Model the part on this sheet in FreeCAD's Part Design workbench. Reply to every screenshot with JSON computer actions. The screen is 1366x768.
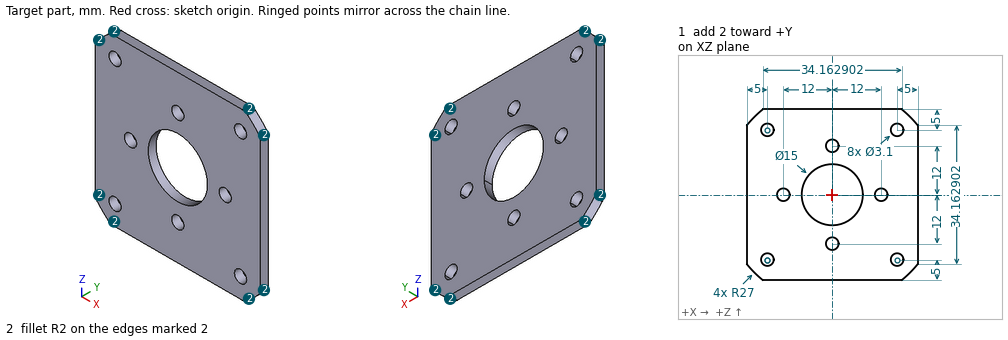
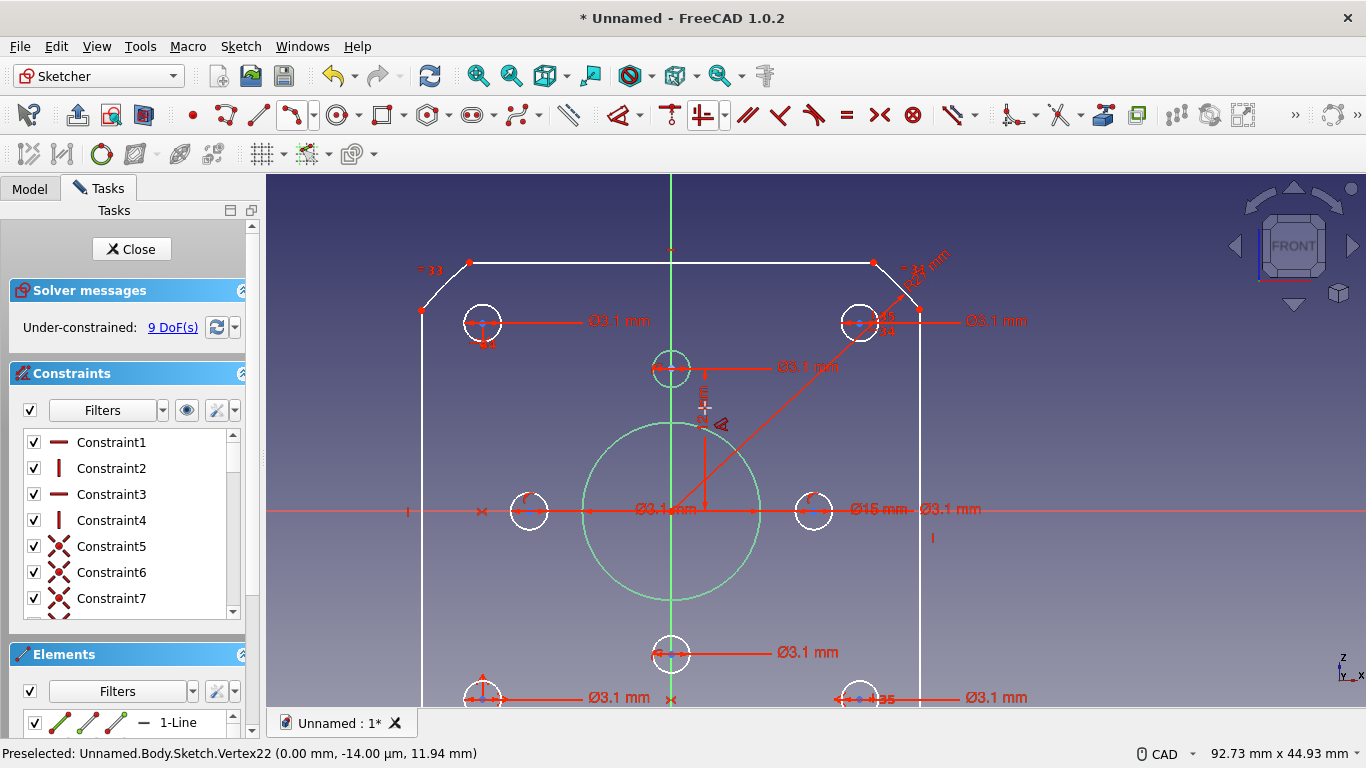
{"action": "left_click", "coordinate": [814, 511]}
{"action": "left_click", "coordinate": [710, 545]}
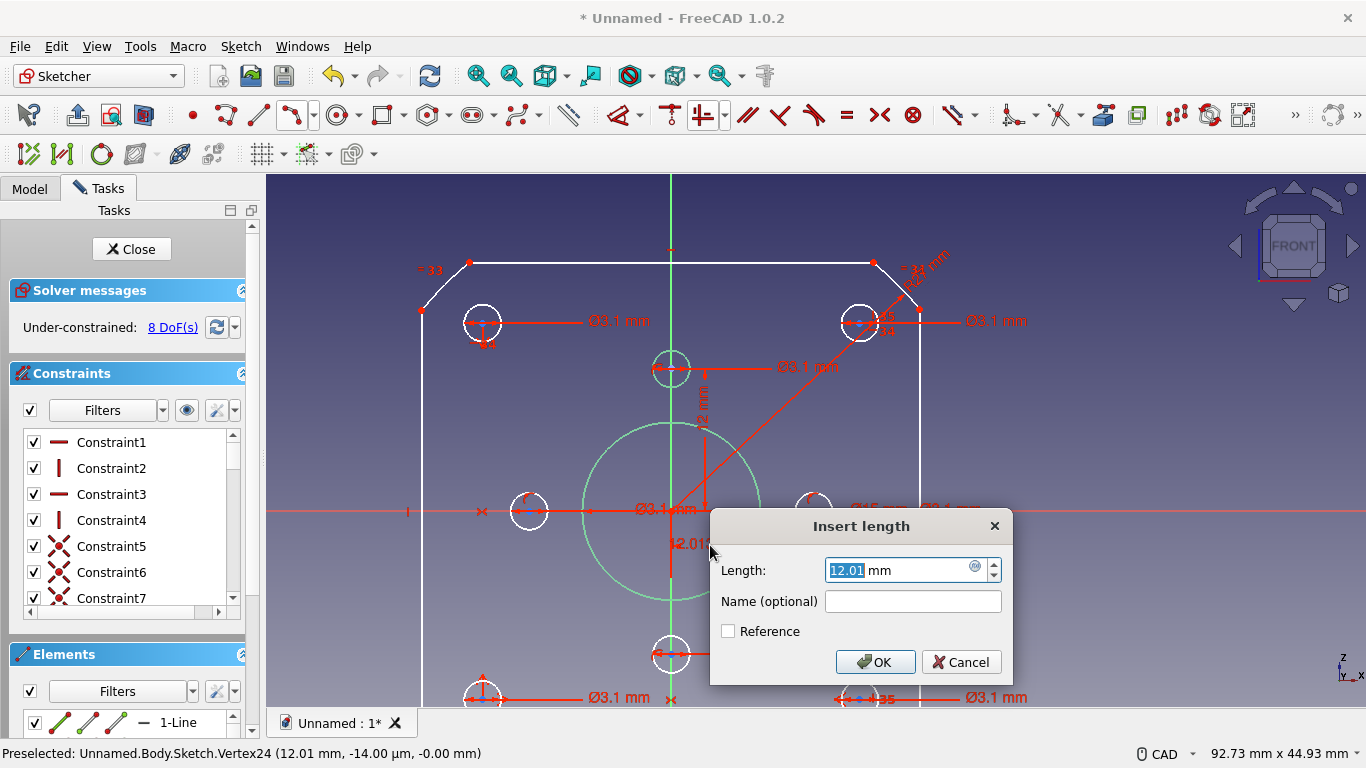
{"action": "type", "text": "12"}
{"action": "key", "text": "Return"}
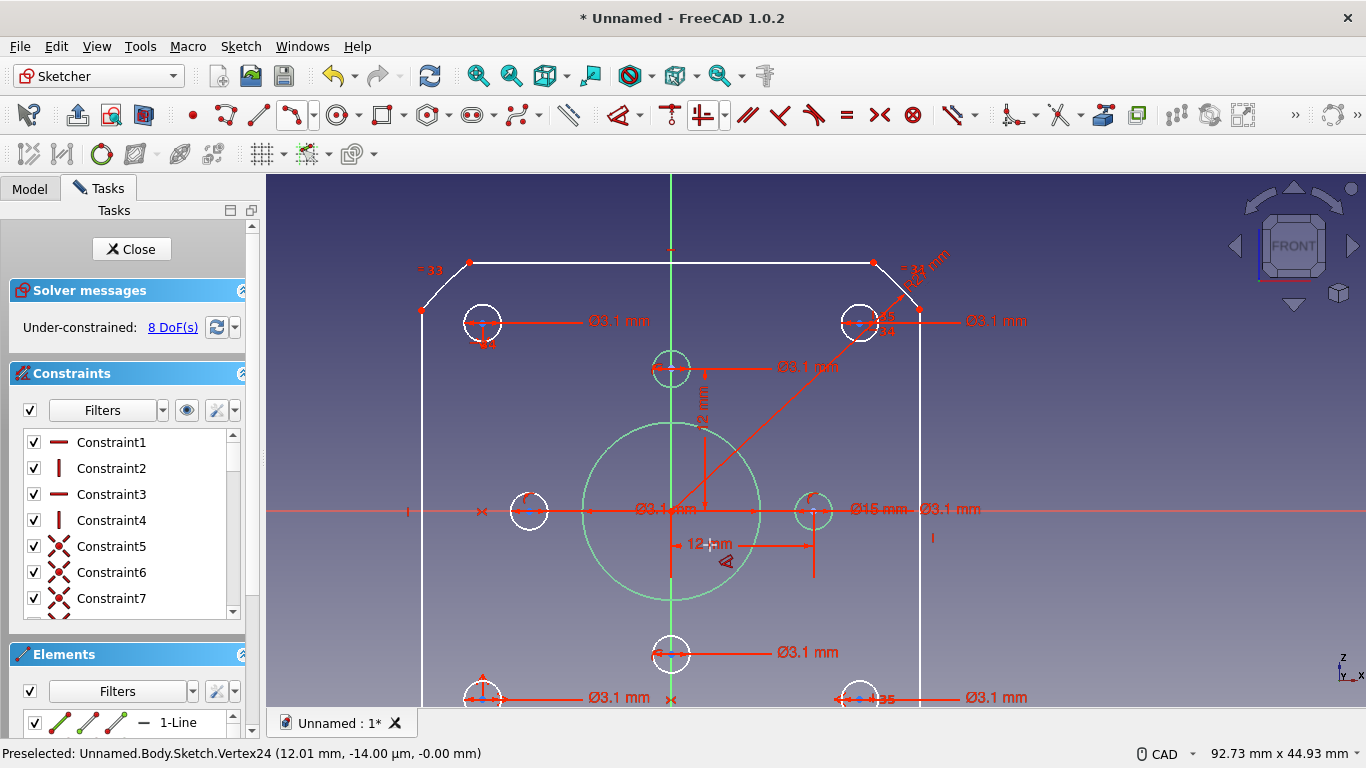
{"action": "left_click", "coordinate": [529, 511]}
{"action": "left_click", "coordinate": [568, 545]}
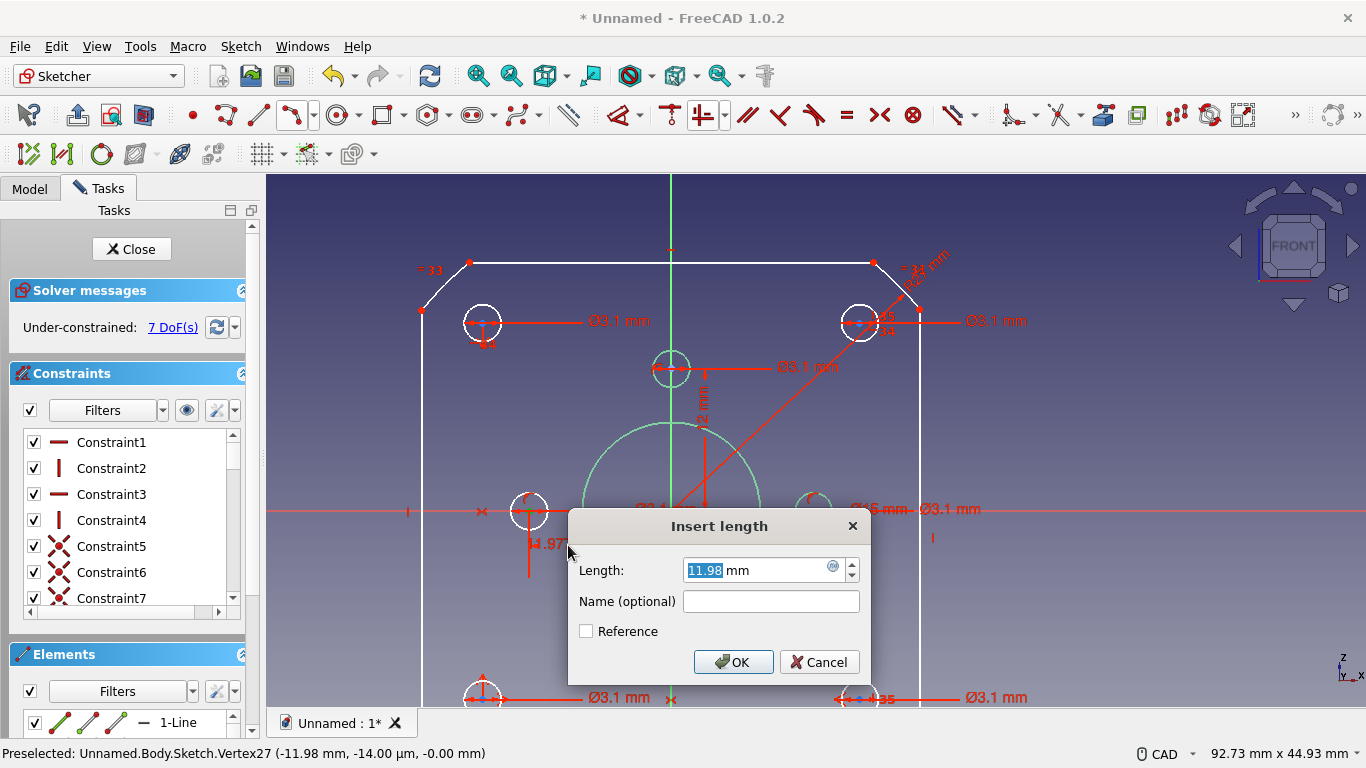
{"action": "type", "text": "12"}
{"action": "key", "text": "Return"}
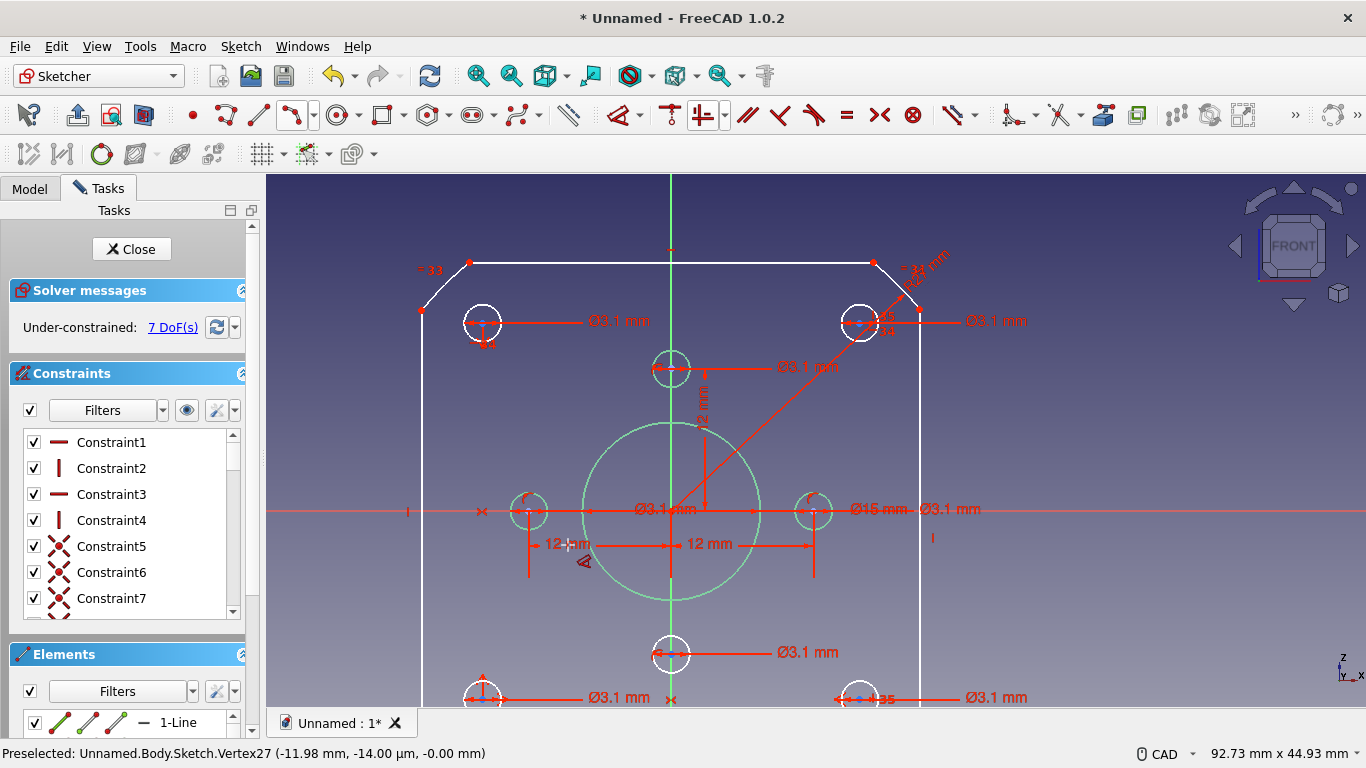
{"action": "left_click", "coordinate": [671, 654]}
{"action": "left_click", "coordinate": [705, 616]}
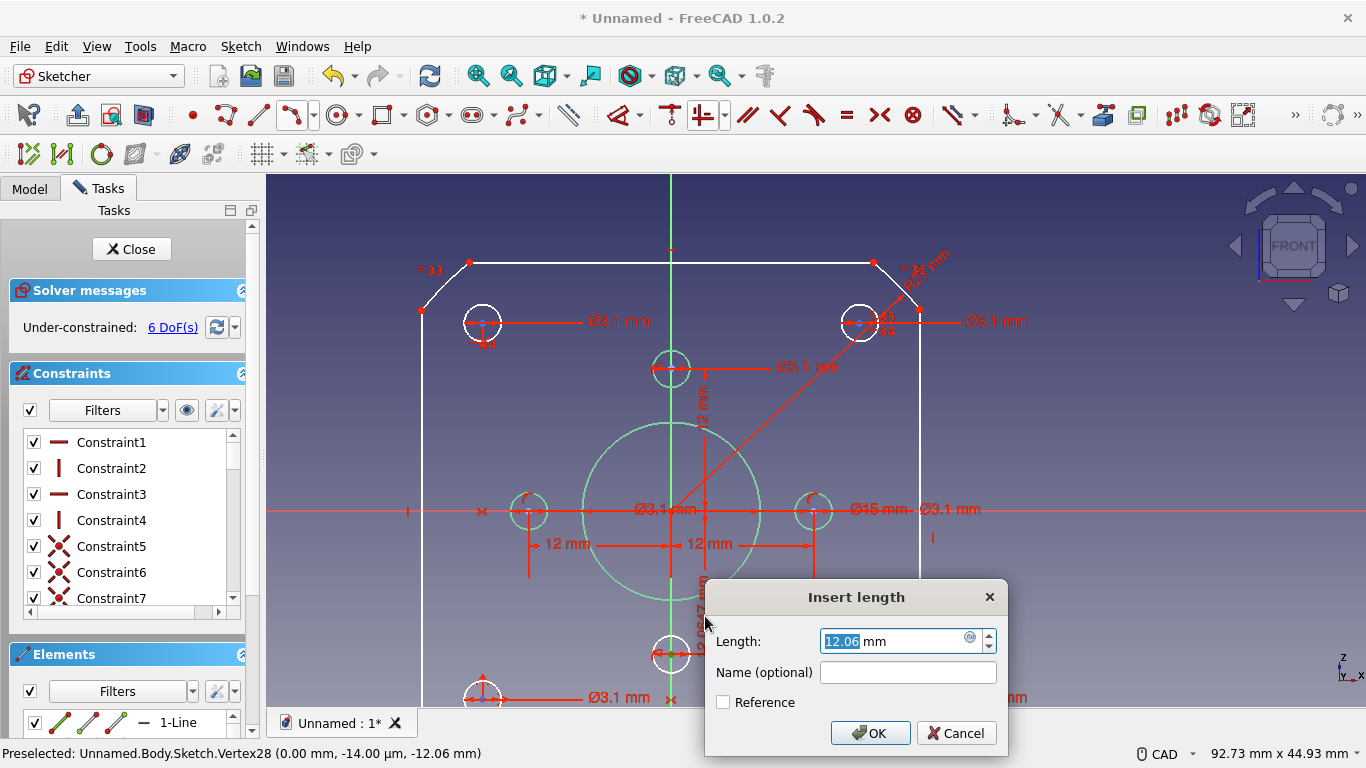
{"action": "type", "text": "12"}
{"action": "key", "text": "Return"}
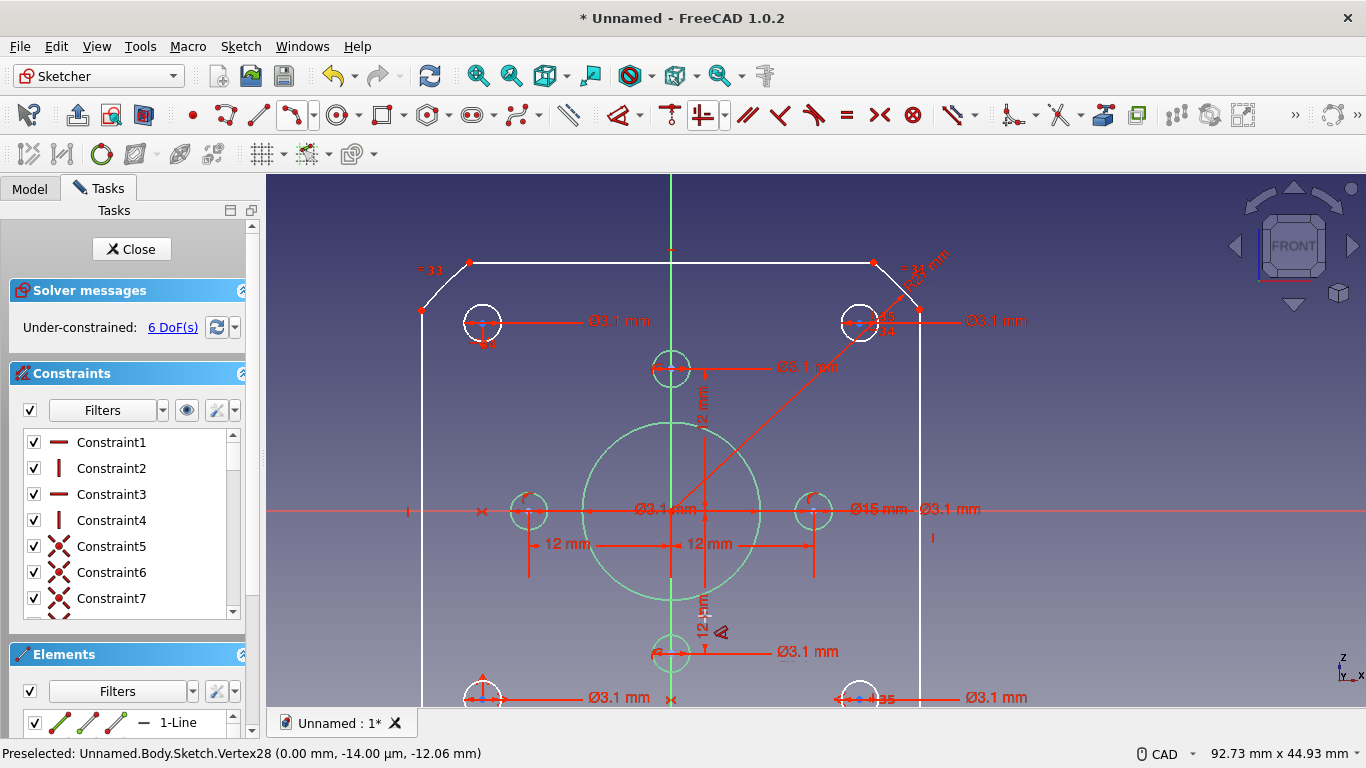
{"action": "left_click", "coordinate": [920, 309]}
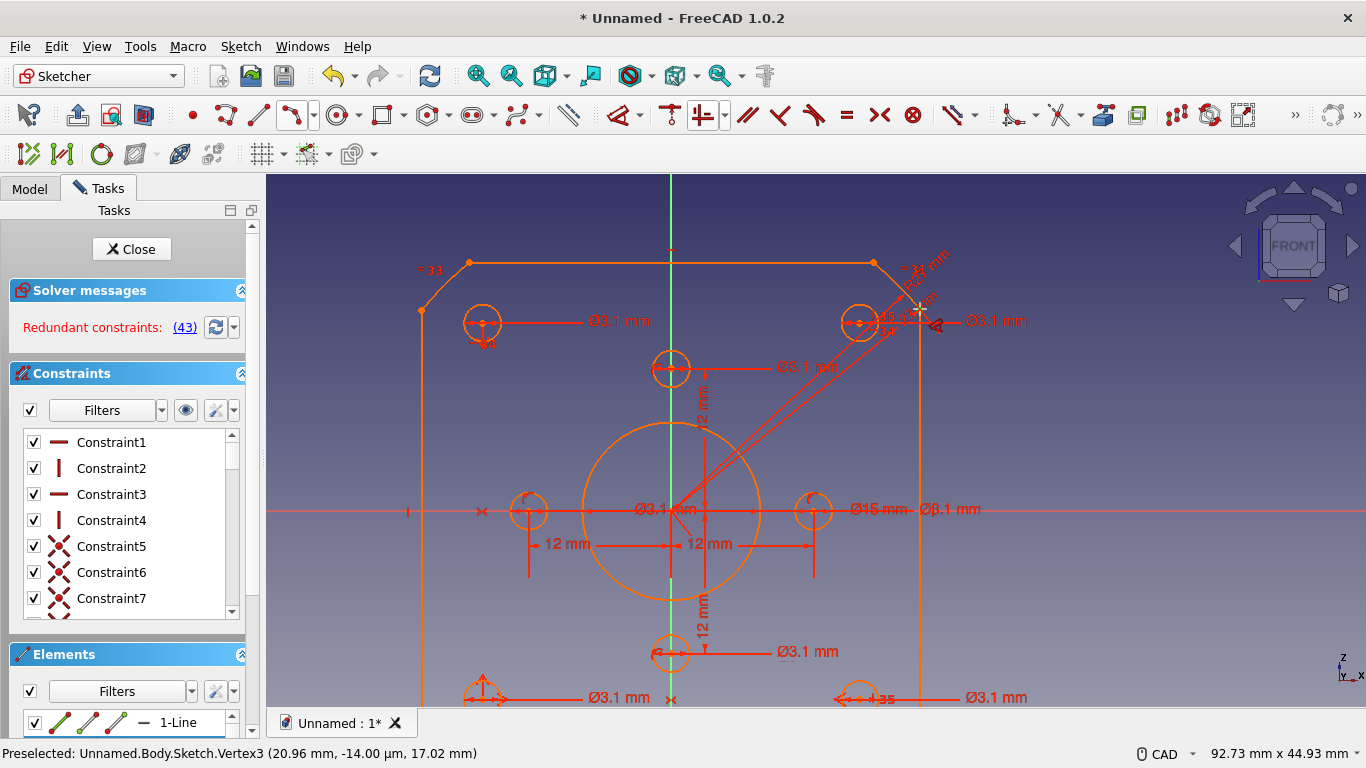
{"action": "left_click", "coordinate": [860, 323]}
{"action": "left_click", "coordinate": [890, 357]}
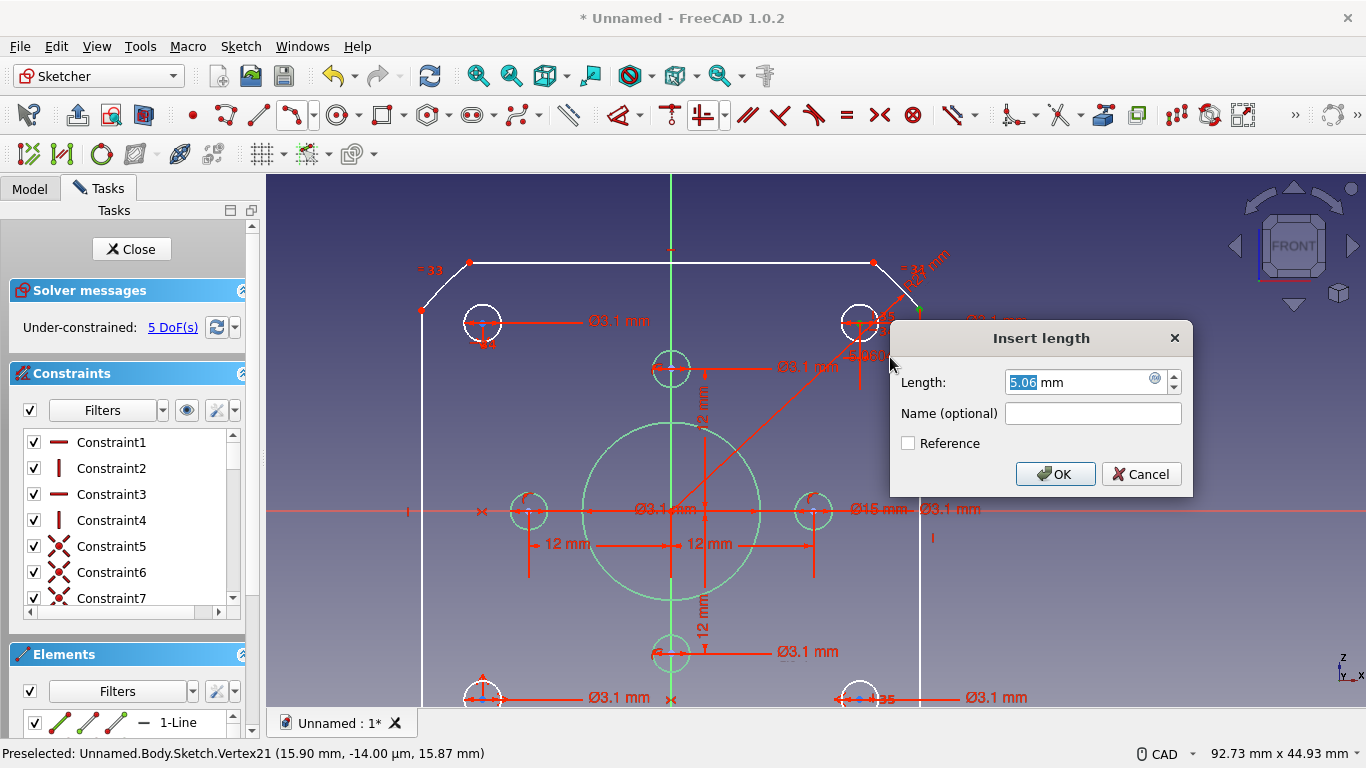
{"action": "type", "text": "5"}
{"action": "key", "text": "Return"}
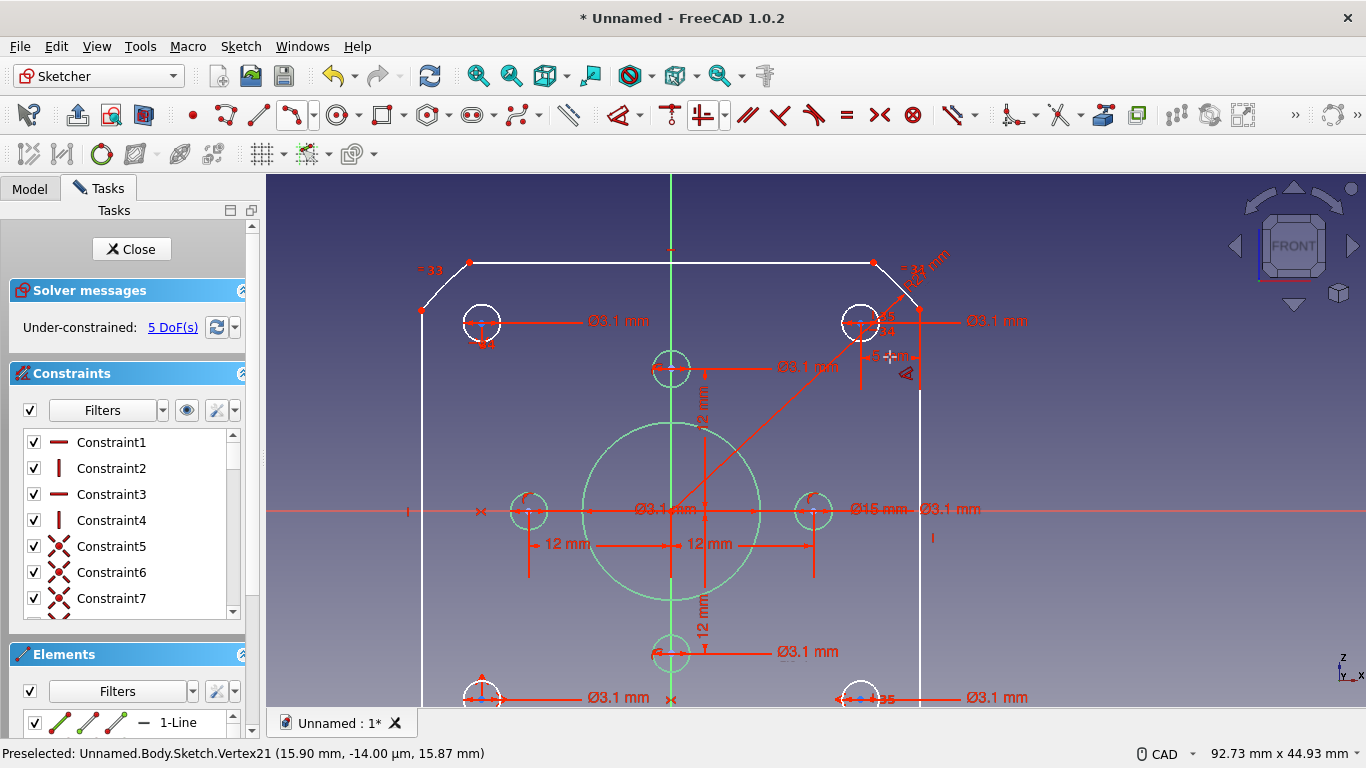
{"action": "left_click", "coordinate": [873, 263]}